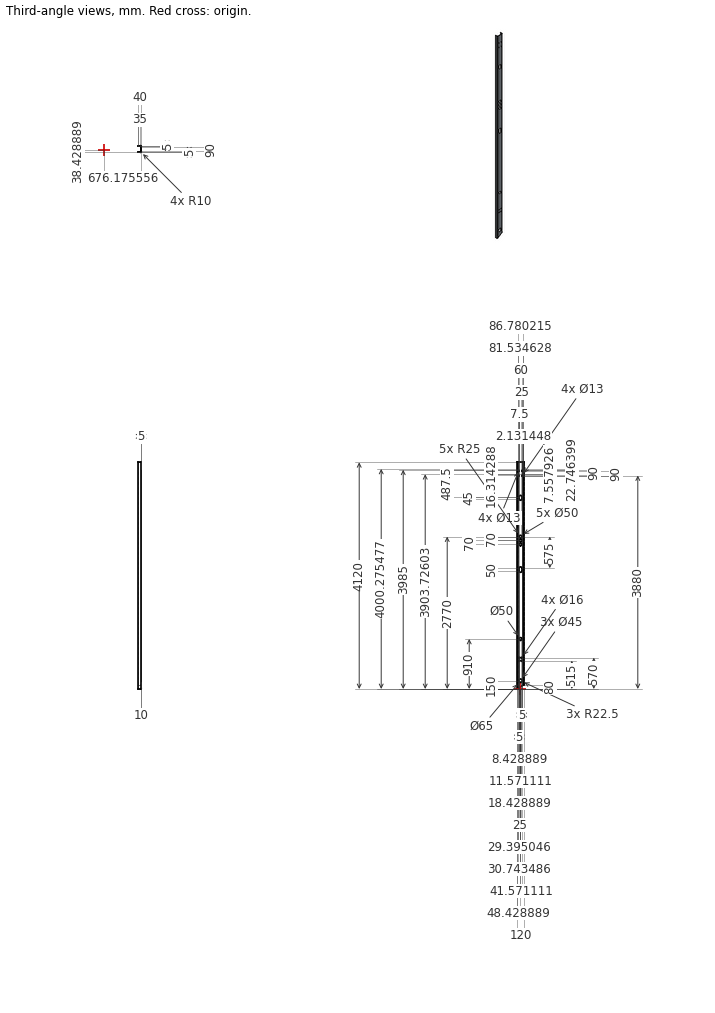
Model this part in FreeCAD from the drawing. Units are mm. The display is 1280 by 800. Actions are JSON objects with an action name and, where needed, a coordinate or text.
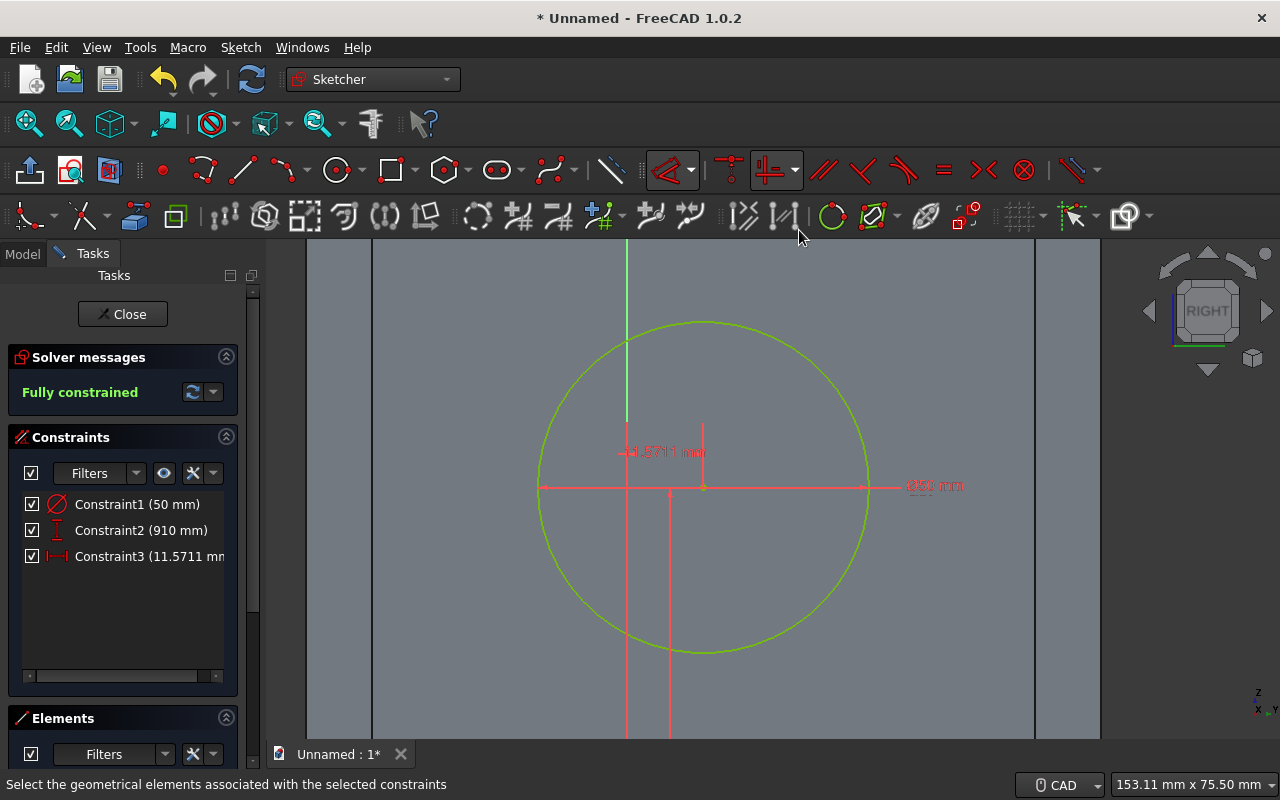
{"action": "left_click", "coordinate": [123, 314]}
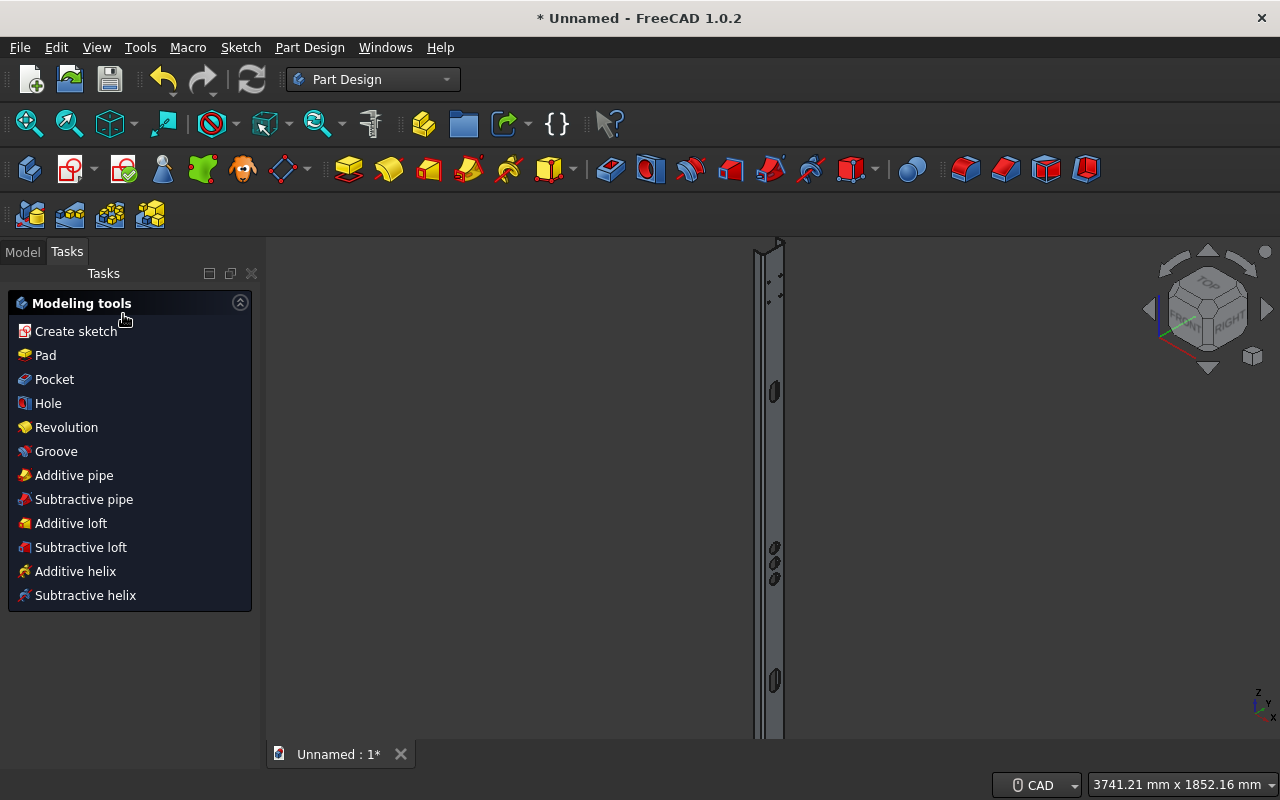
{"action": "left_click", "coordinate": [612, 170]}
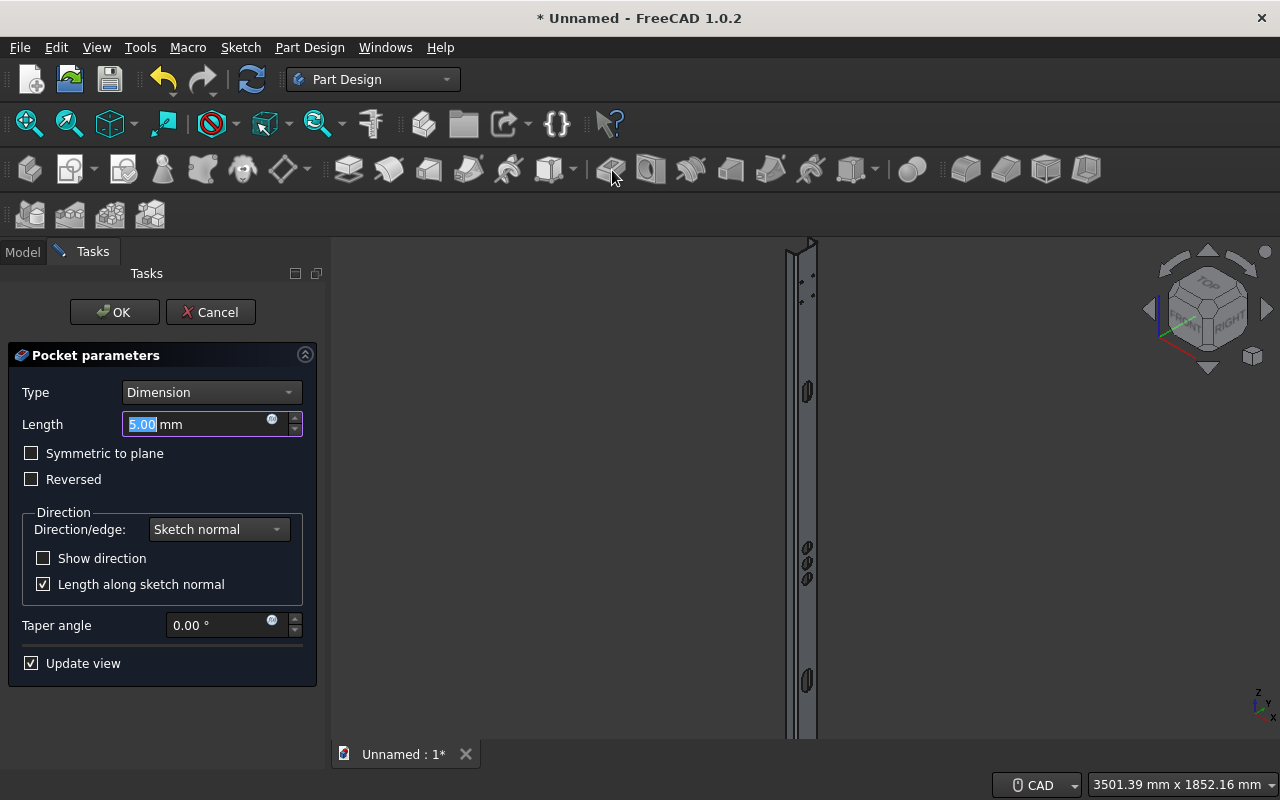
{"action": "type", "text": "10"}
{"action": "key", "text": "Tab"}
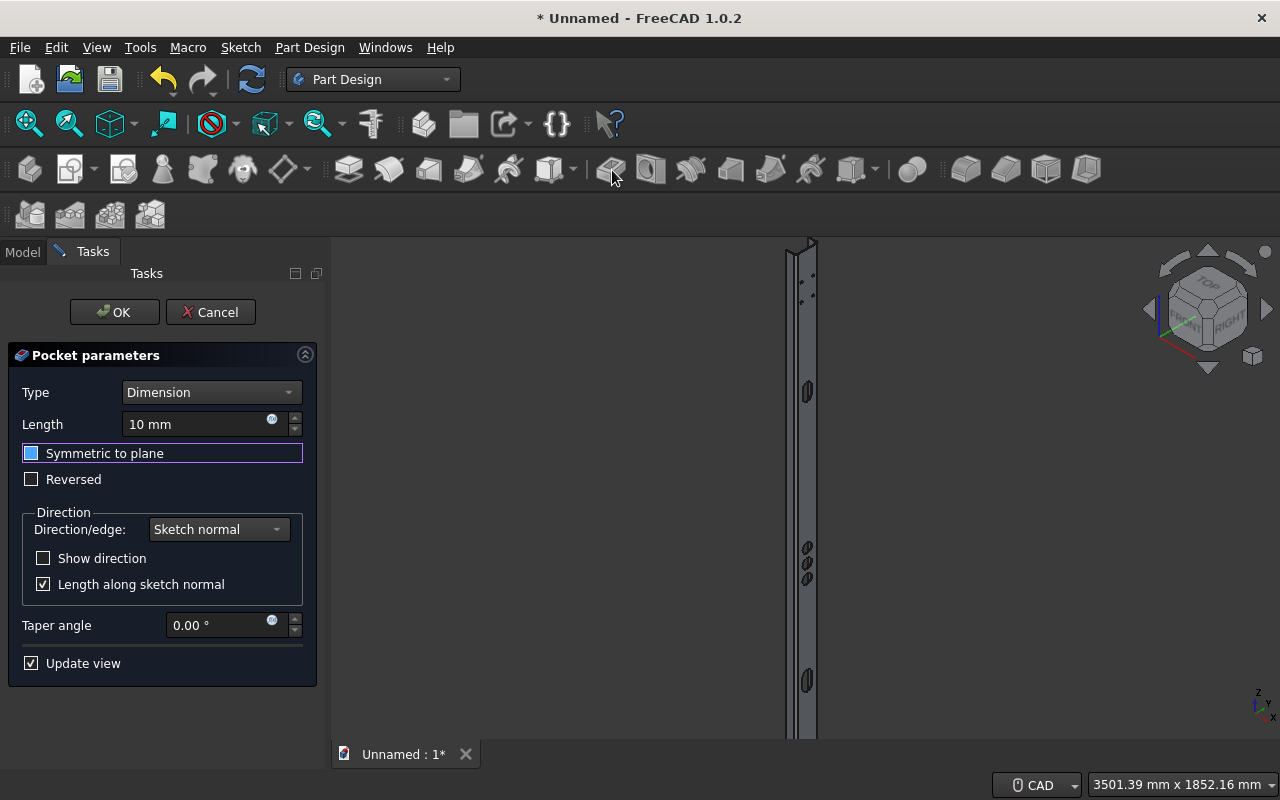
{"action": "left_click", "coordinate": [115, 312]}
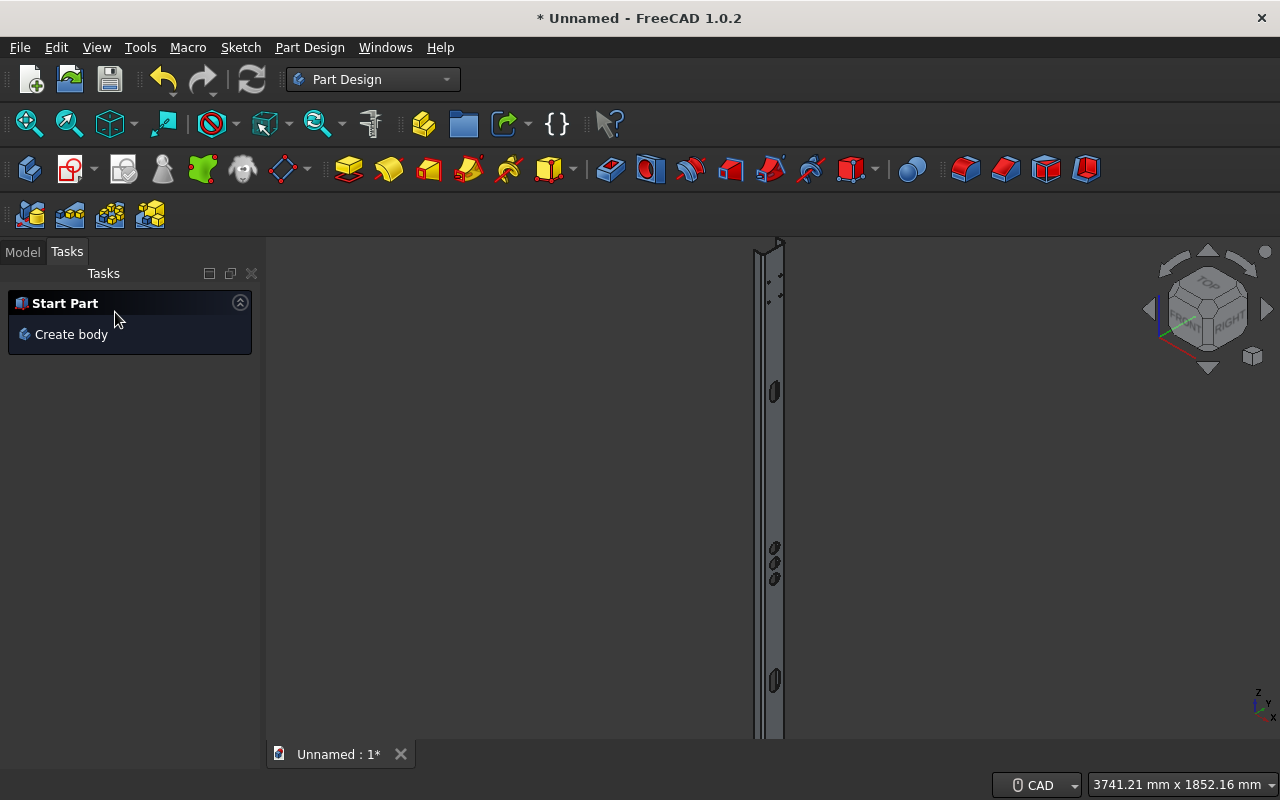
{"action": "key", "text": "v f"}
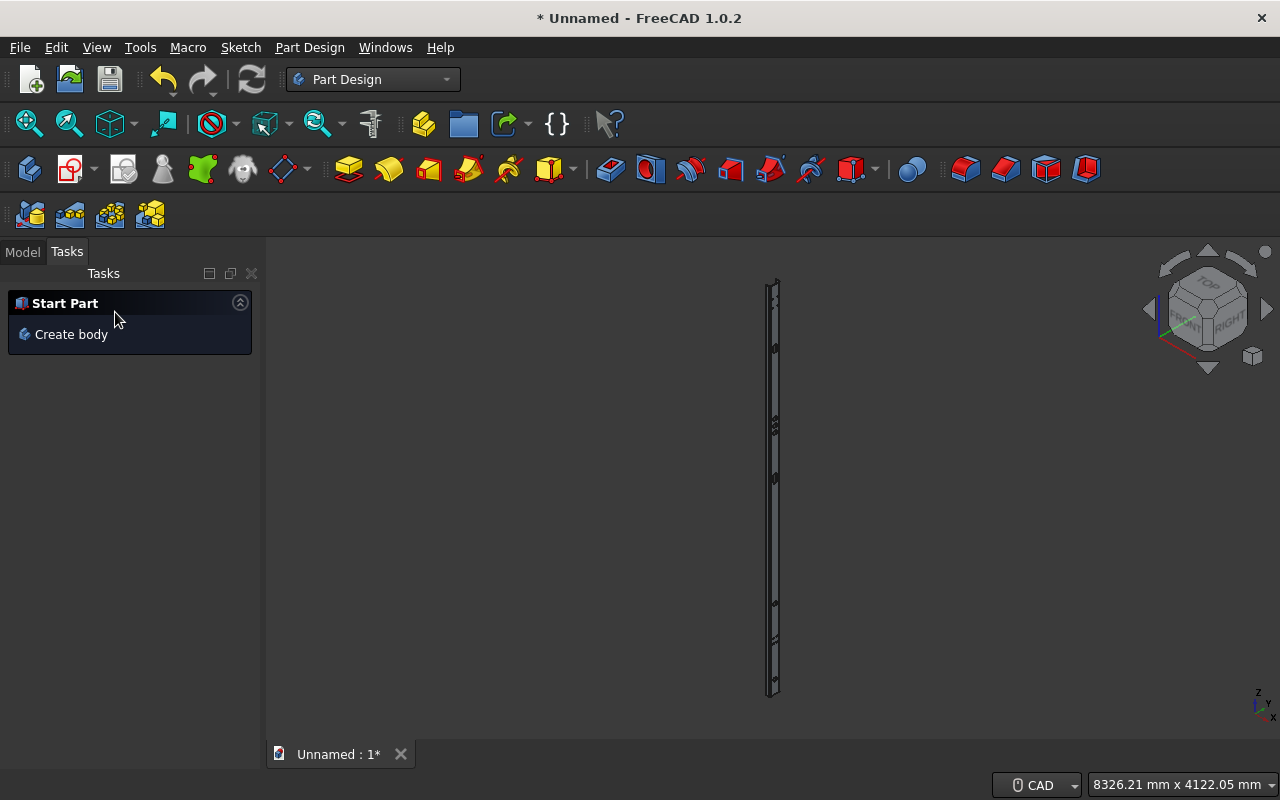
{"action": "scroll", "coordinate": [775, 313], "scroll_direction": "up", "scroll_amount": 4}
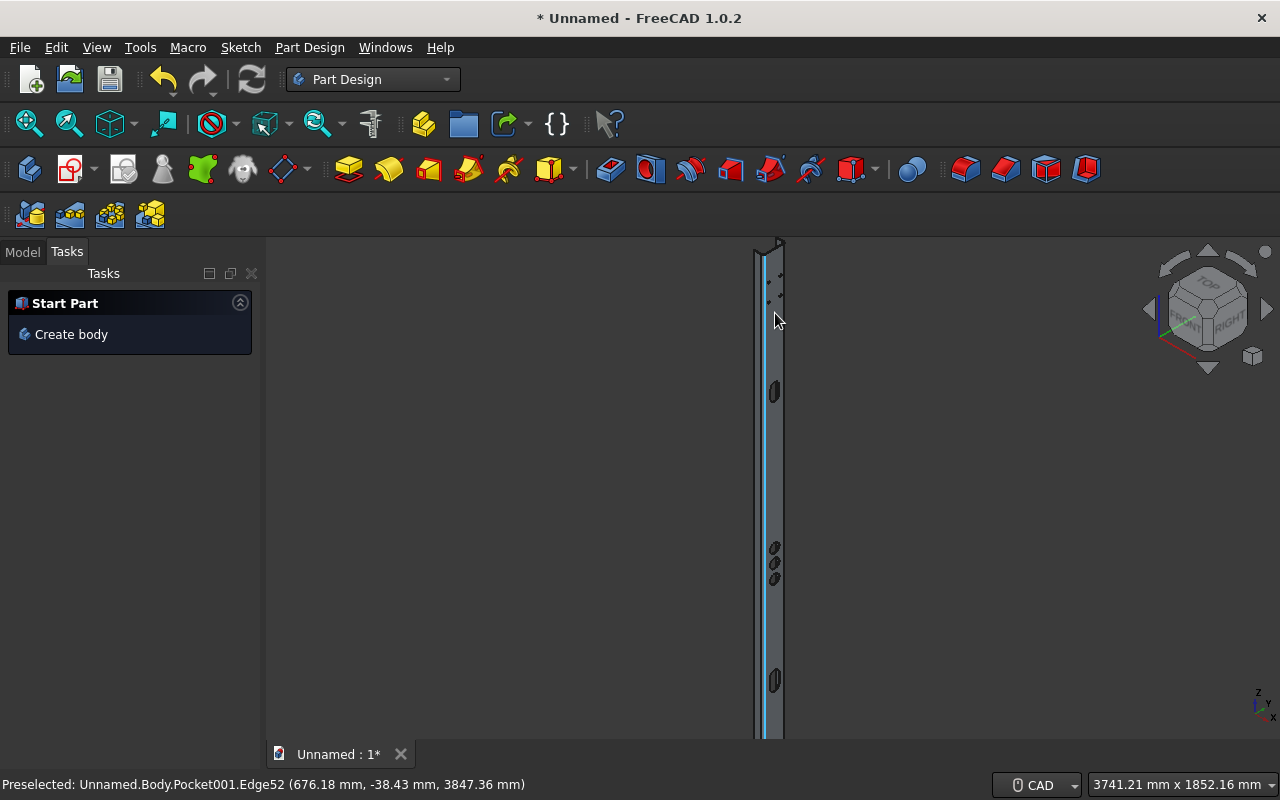
{"action": "left_click", "coordinate": [775, 313]}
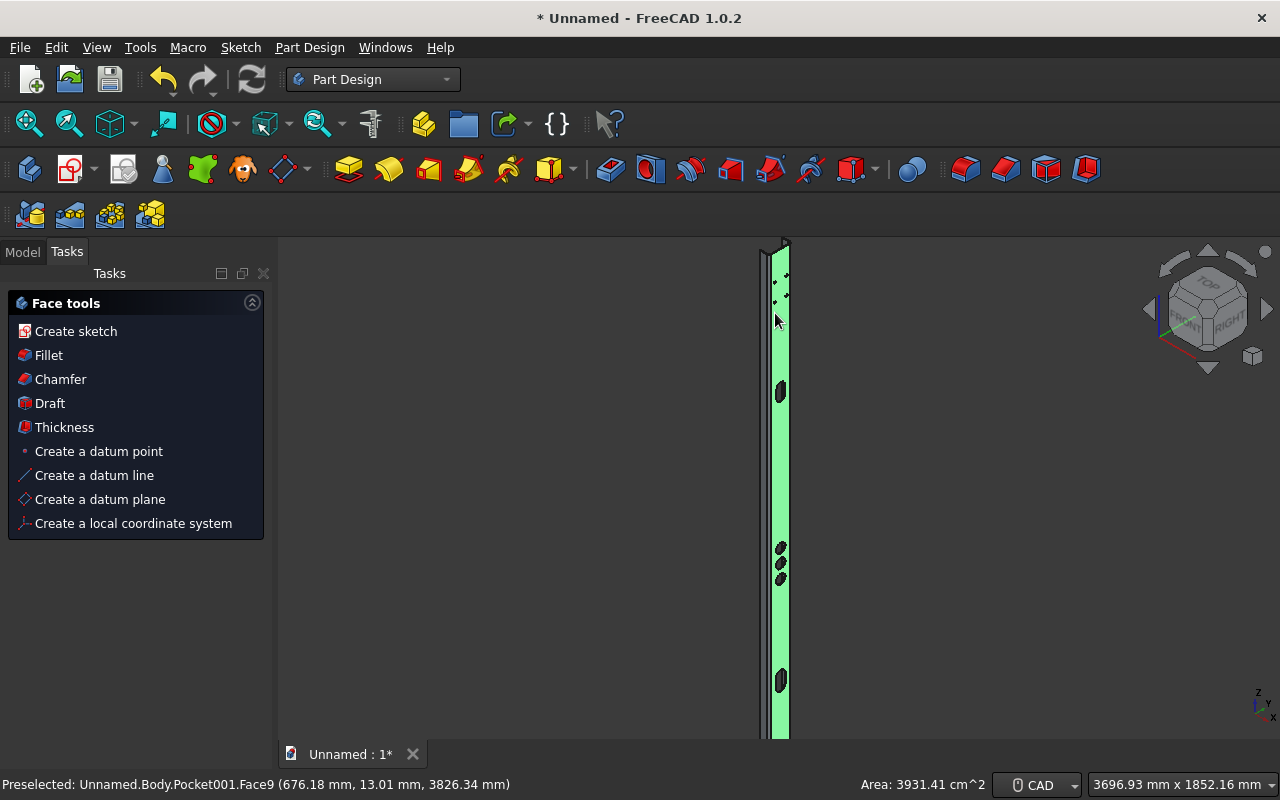
{"action": "left_click", "coordinate": [70, 170]}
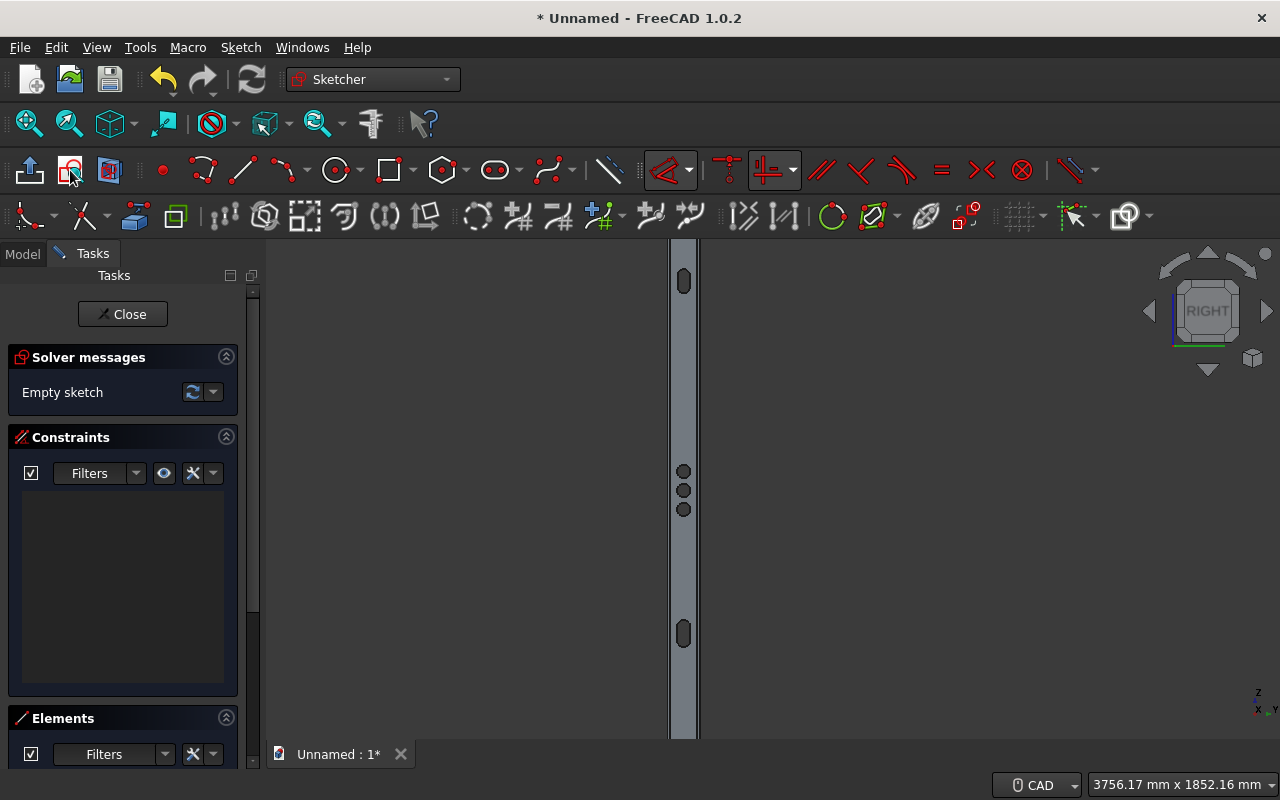
{"action": "scroll", "coordinate": [704, 489], "scroll_direction": "down", "scroll_amount": 5}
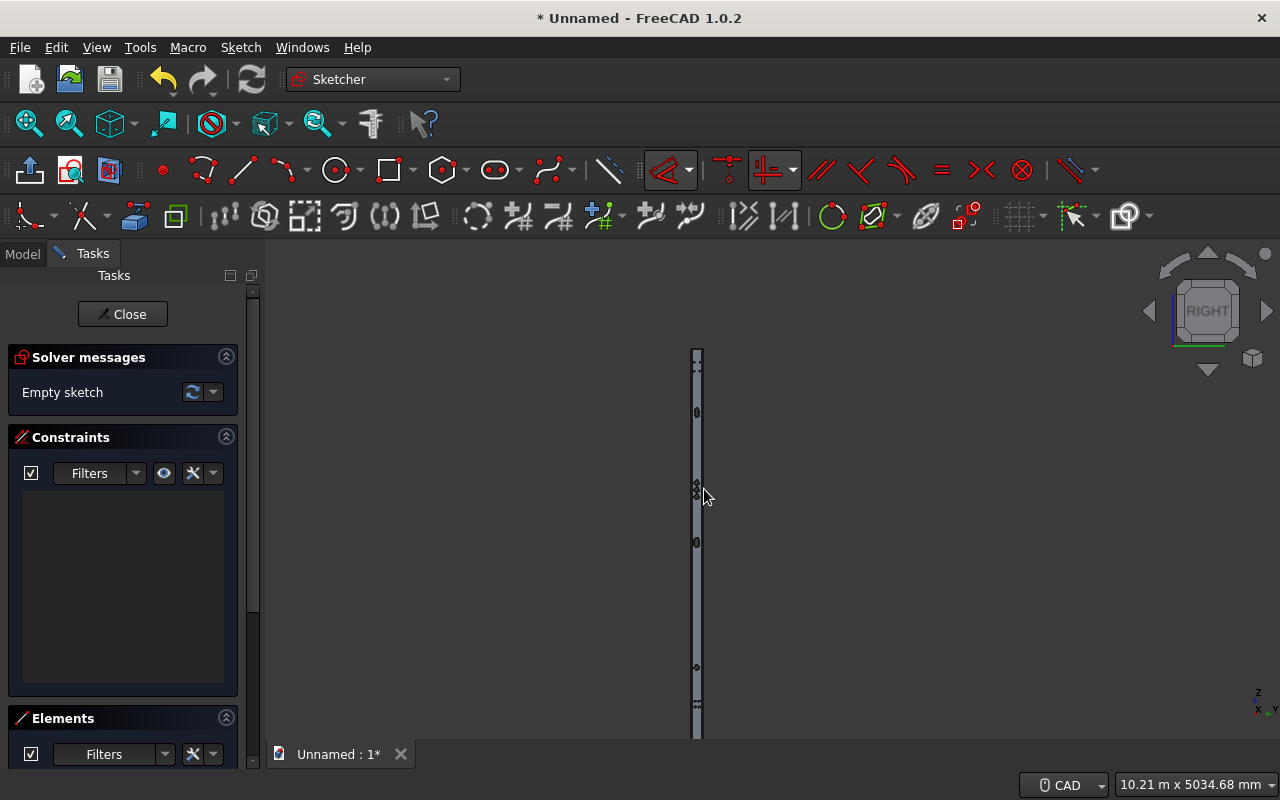
{"action": "scroll", "coordinate": [696, 362], "scroll_direction": "up", "scroll_amount": 15}